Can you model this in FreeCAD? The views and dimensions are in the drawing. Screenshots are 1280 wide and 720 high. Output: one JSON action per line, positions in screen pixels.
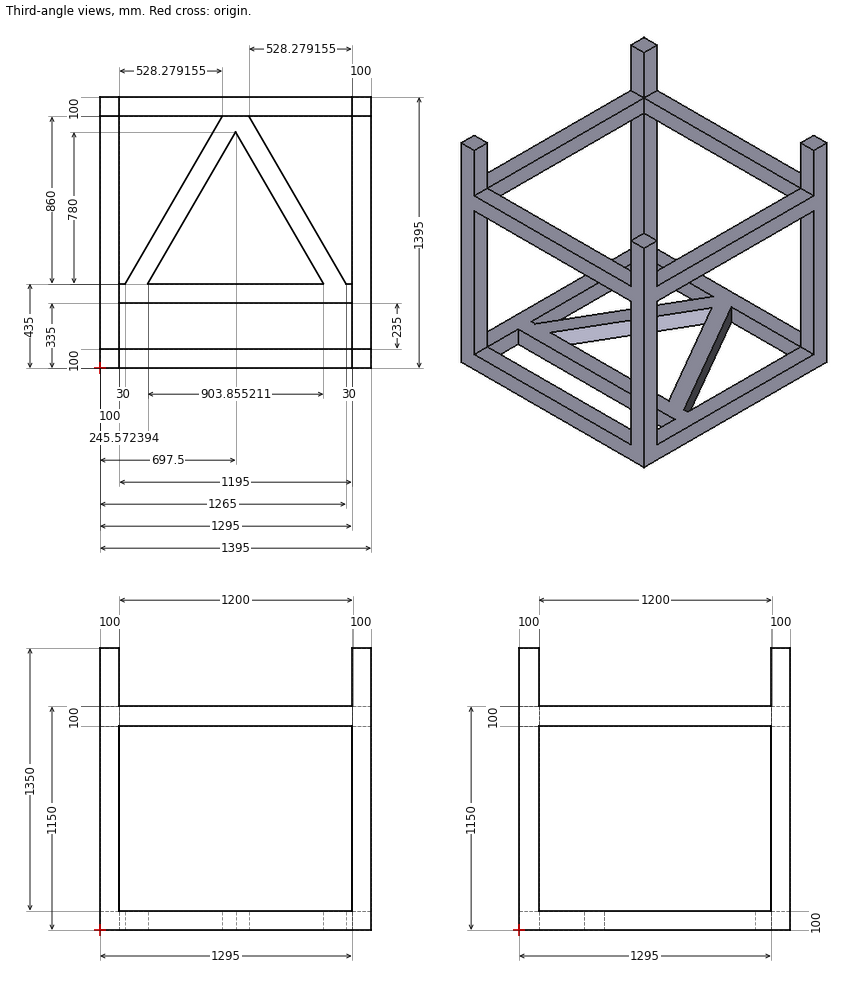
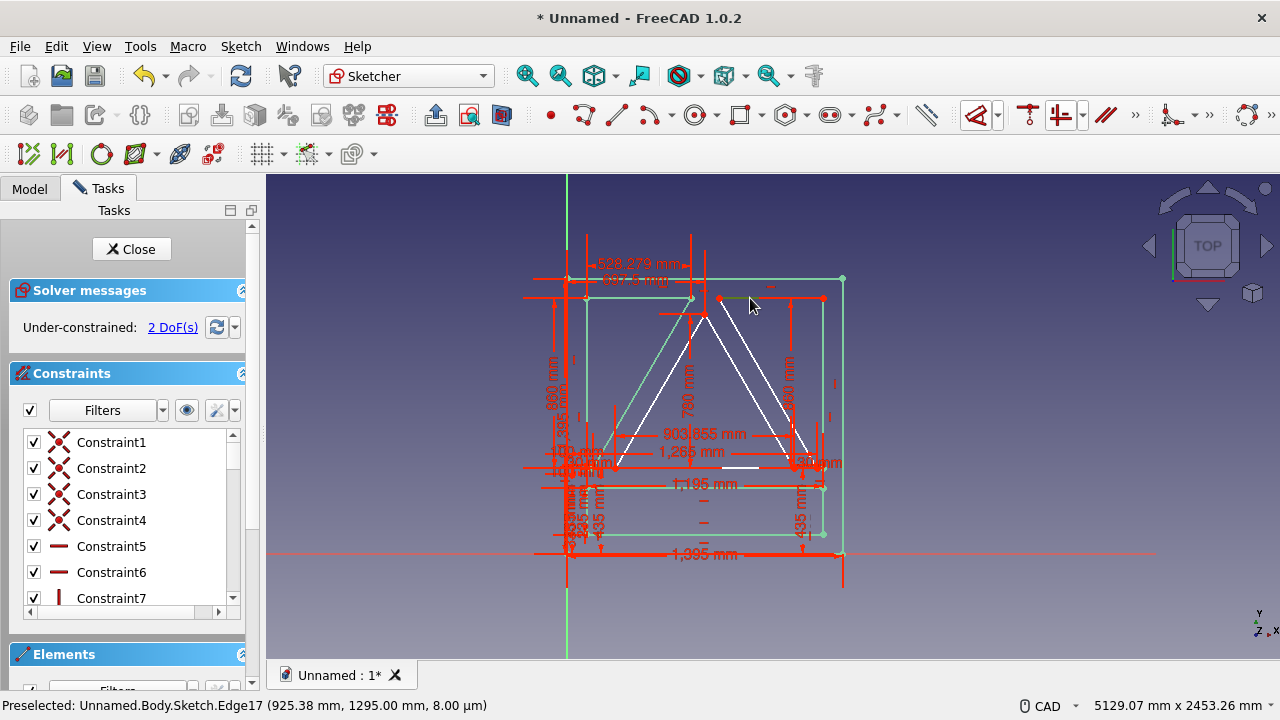
{"action": "key", "text": "l"}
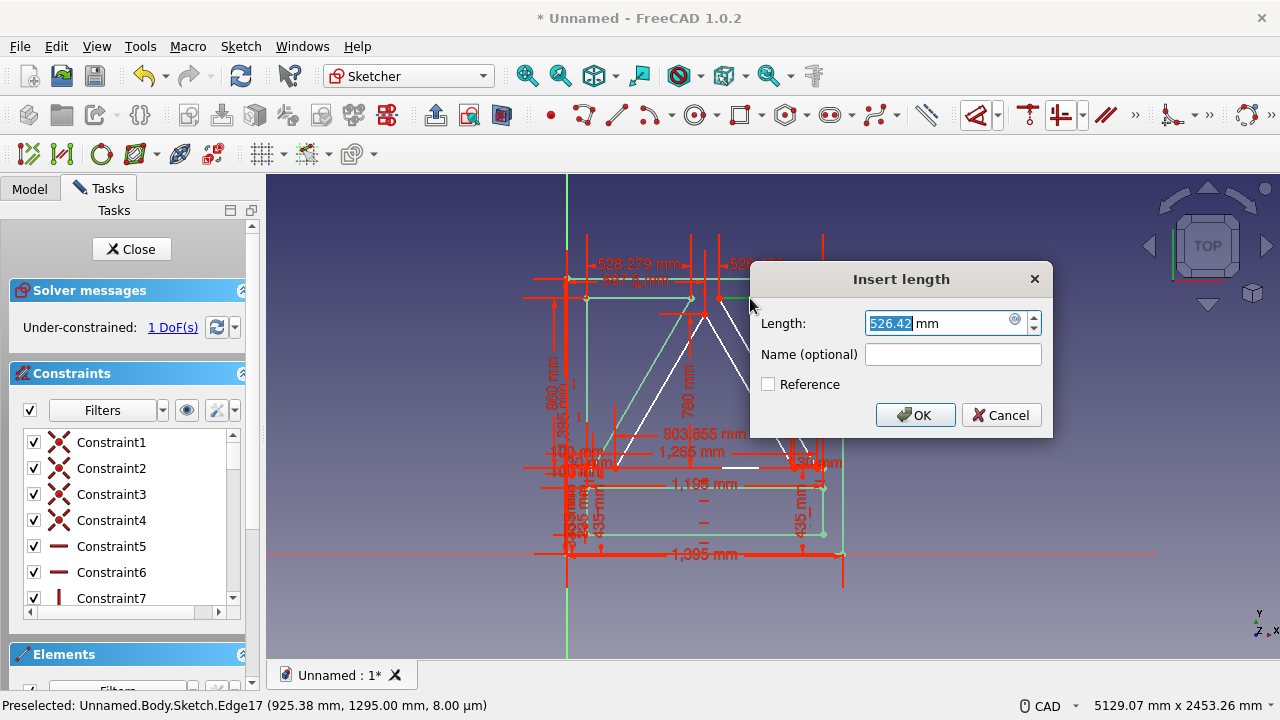
{"action": "type", "text": "528.279155"}
{"action": "key", "text": "Return"}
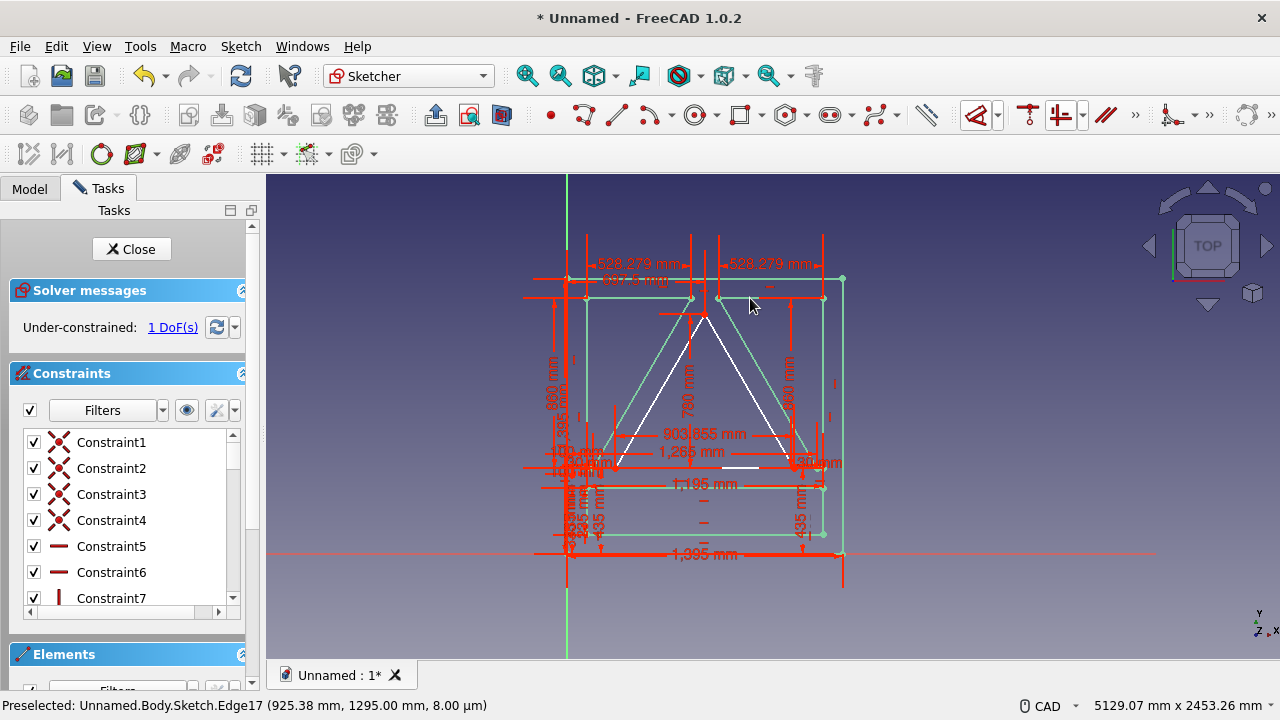
{"action": "left_click", "coordinate": [615, 468]}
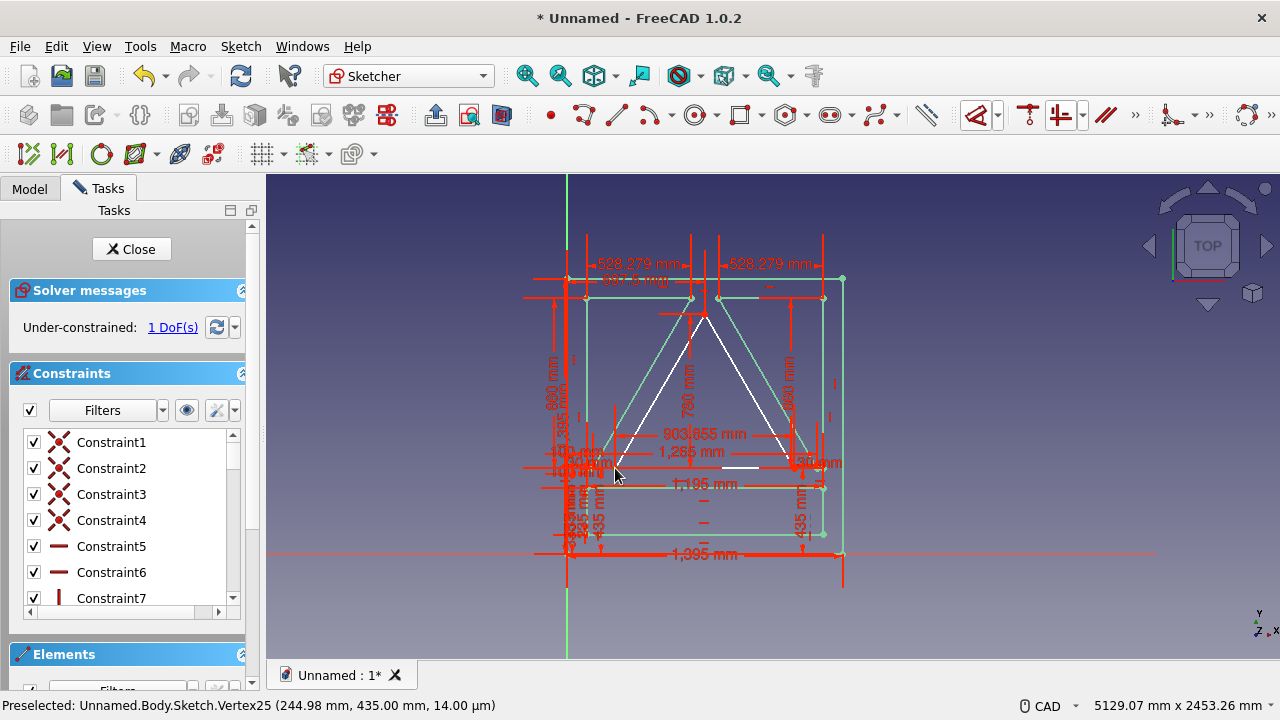
{"action": "left_click", "coordinate": [998, 116]}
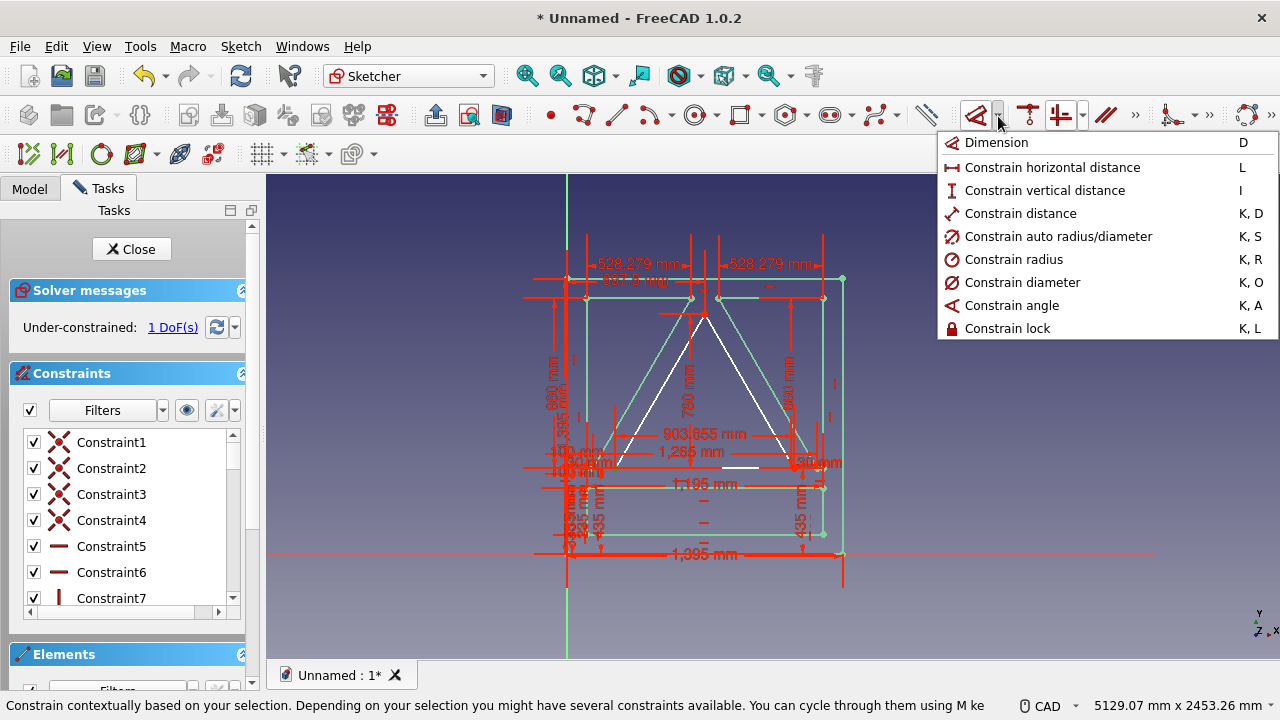
{"action": "left_click", "coordinate": [1108, 168]}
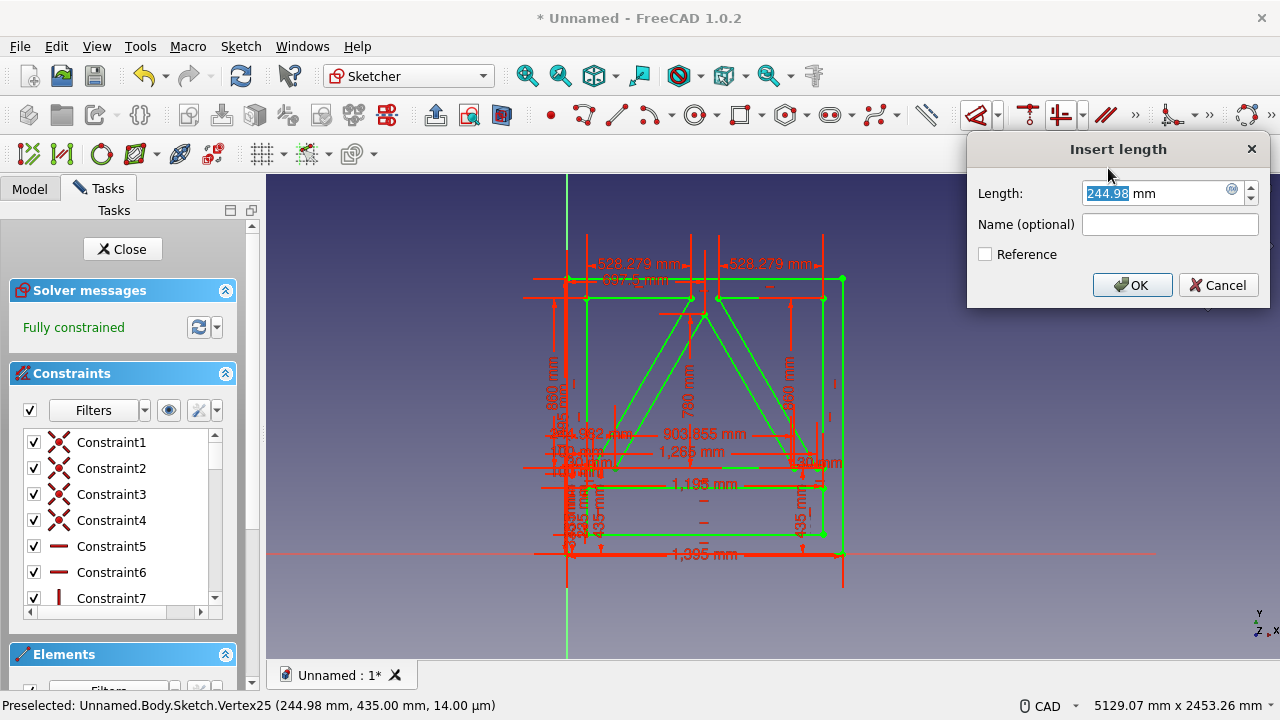
{"action": "type", "text": "245.572394"}
{"action": "key", "text": "Return"}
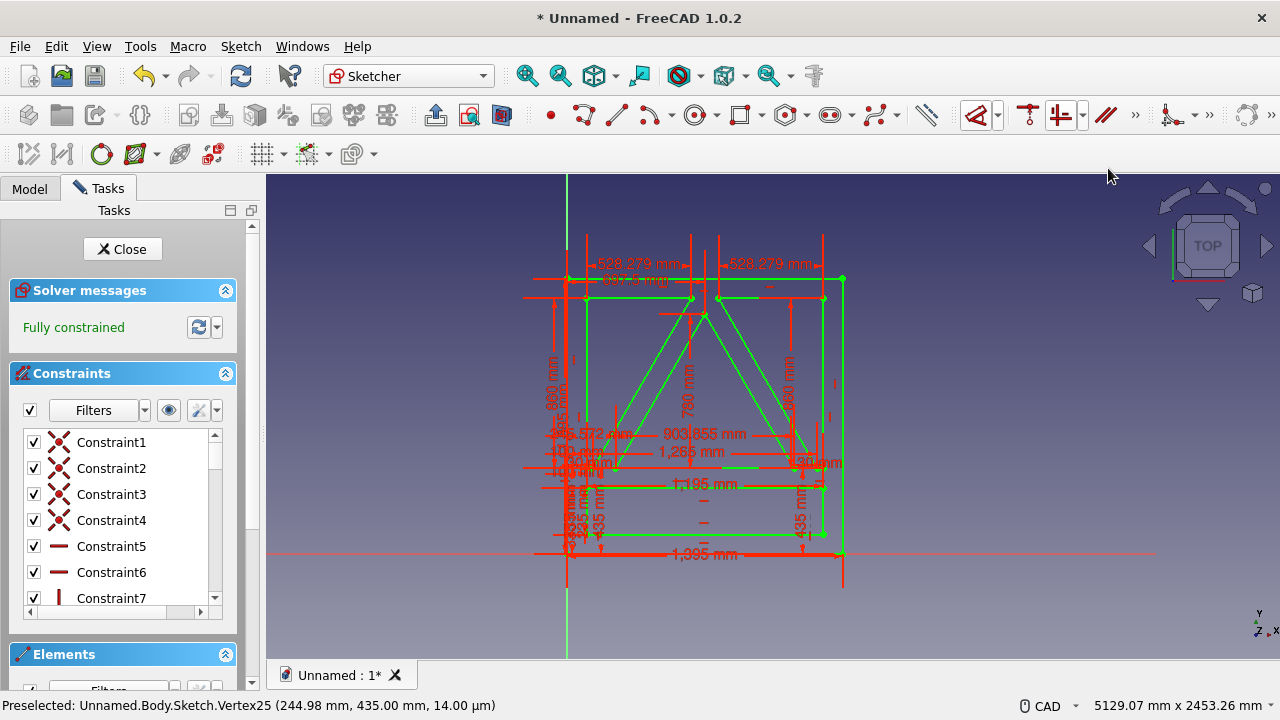
{"action": "left_click", "coordinate": [123, 249]}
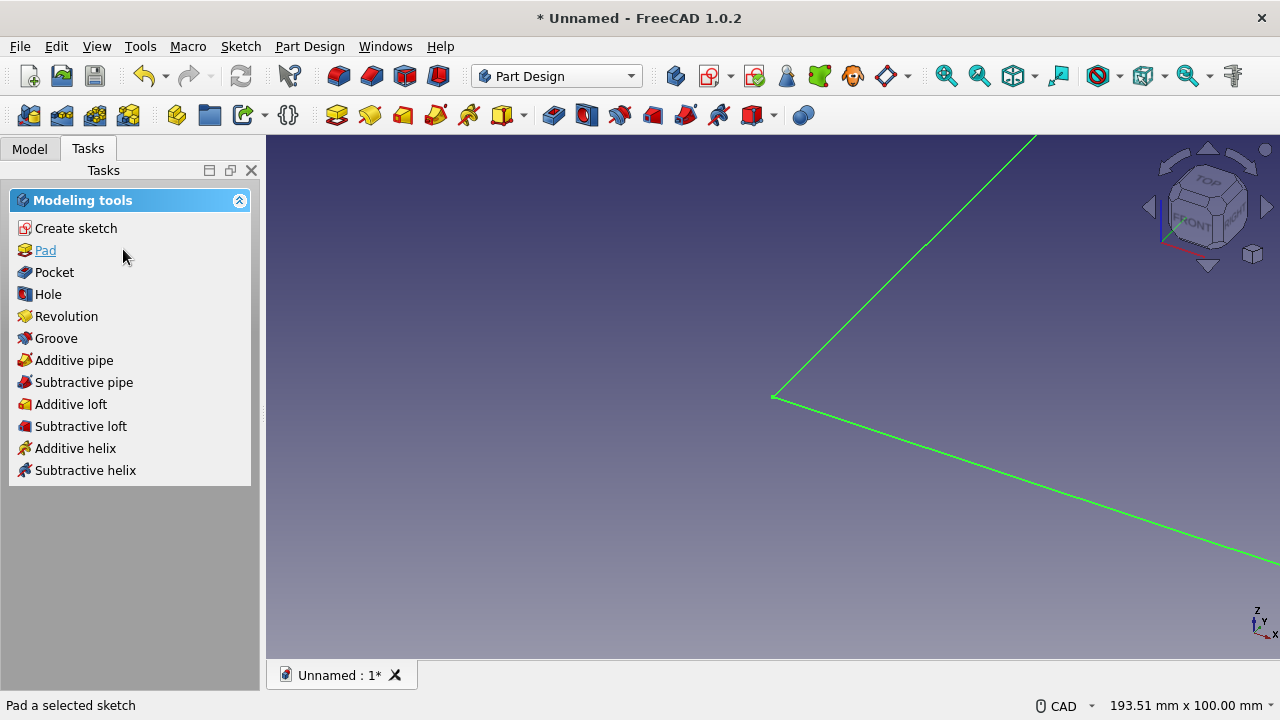
{"action": "left_click", "coordinate": [337, 116]}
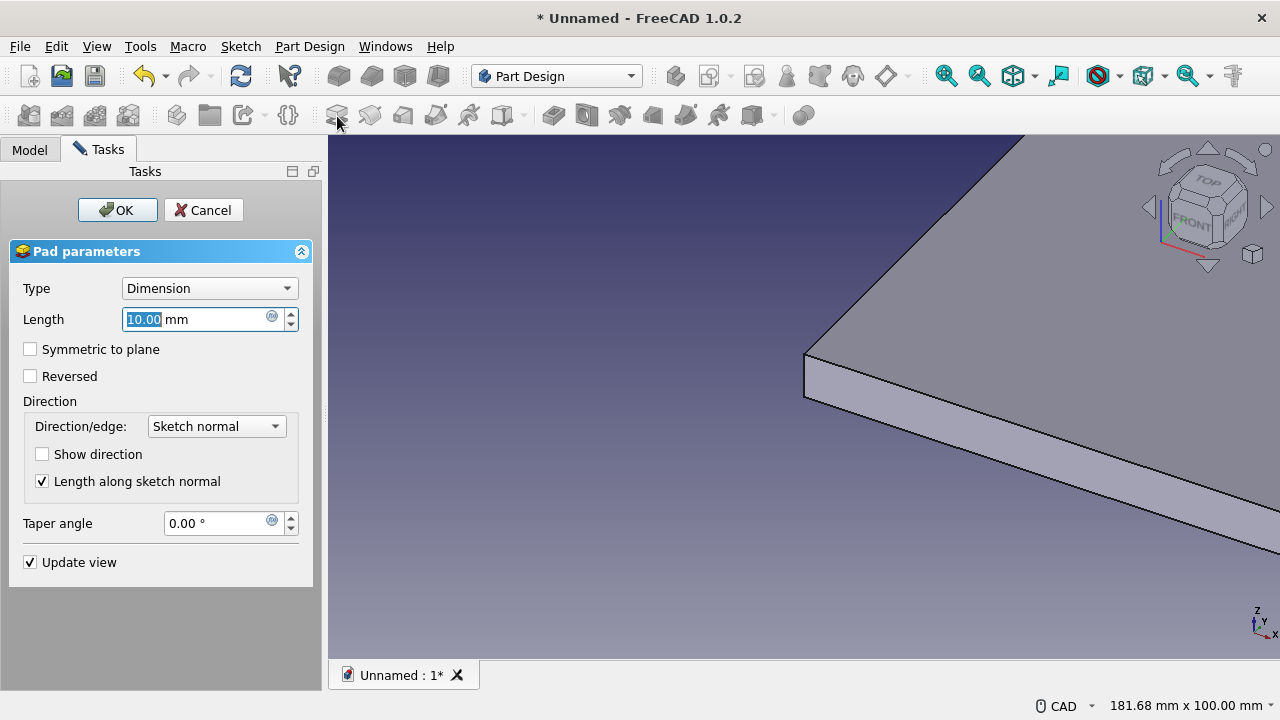
{"action": "type", "text": "100"}
{"action": "key", "text": "Tab"}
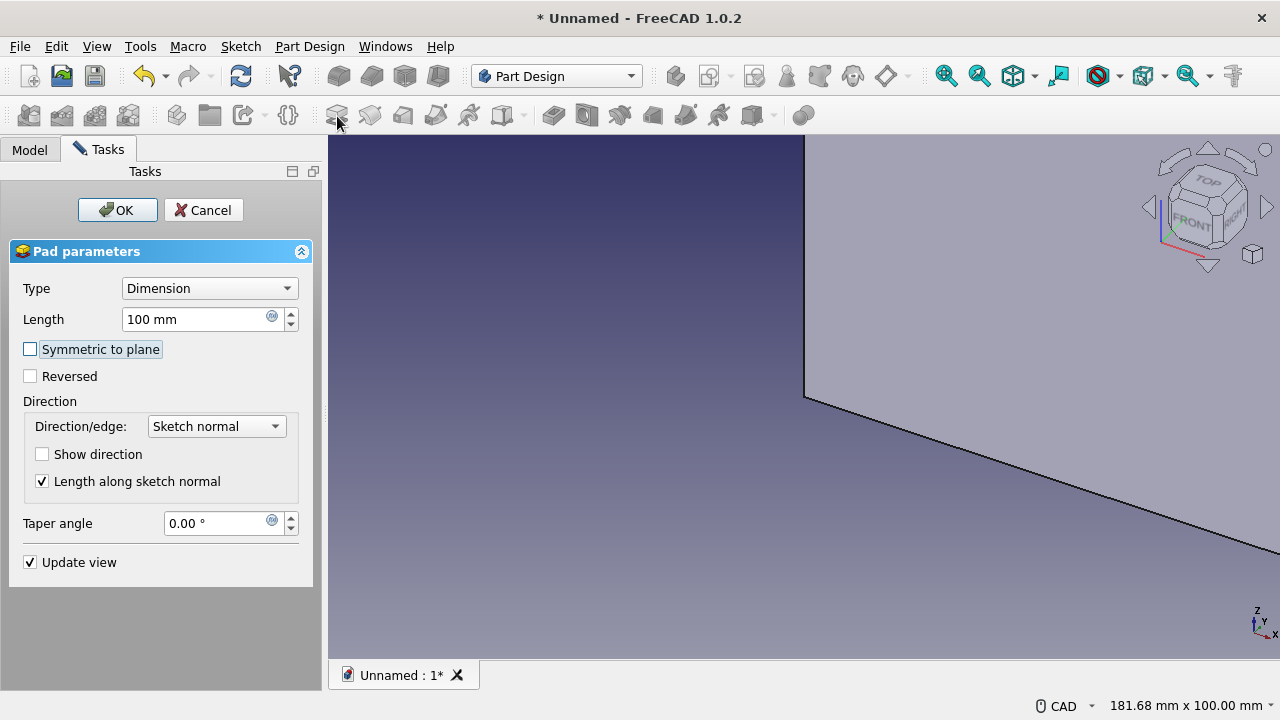
{"action": "left_click", "coordinate": [118, 210]}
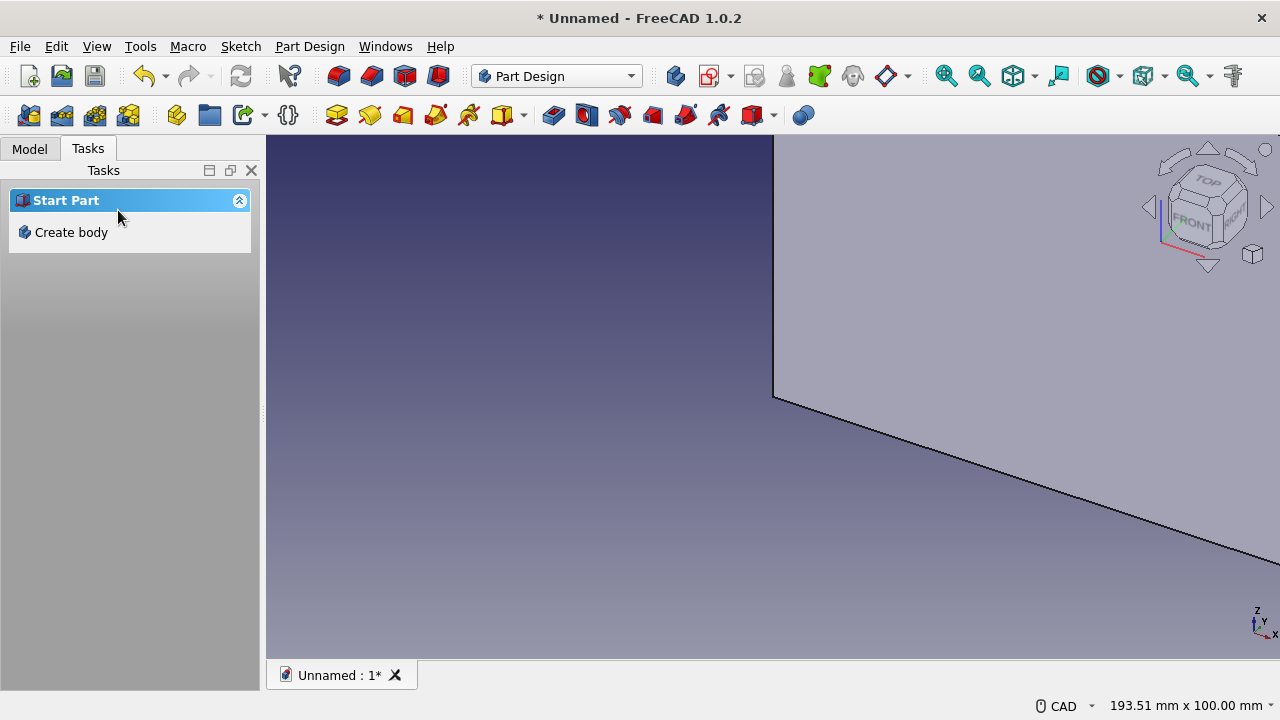
{"action": "left_click", "coordinate": [947, 76]}